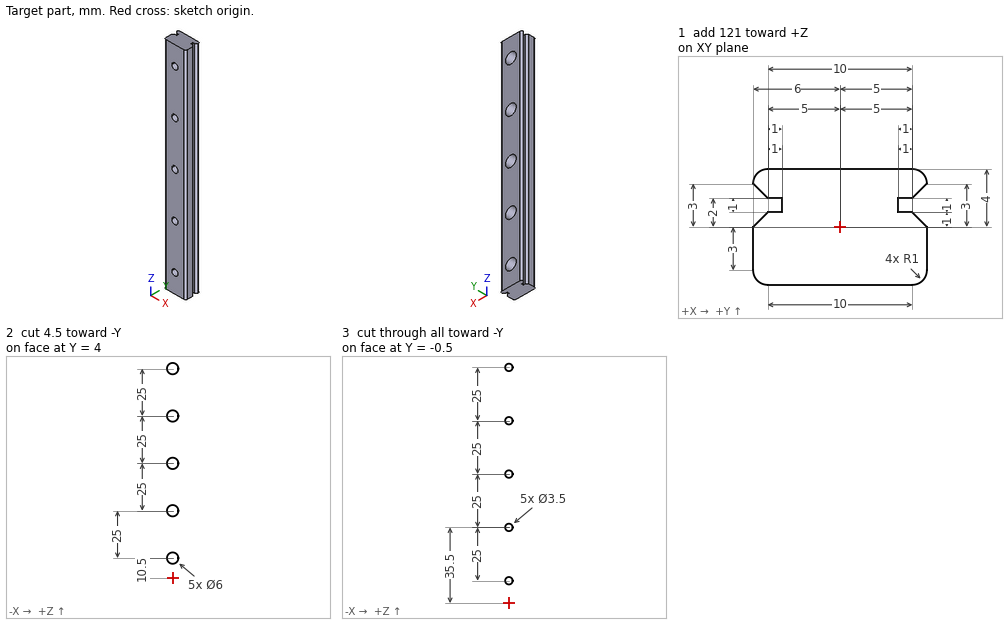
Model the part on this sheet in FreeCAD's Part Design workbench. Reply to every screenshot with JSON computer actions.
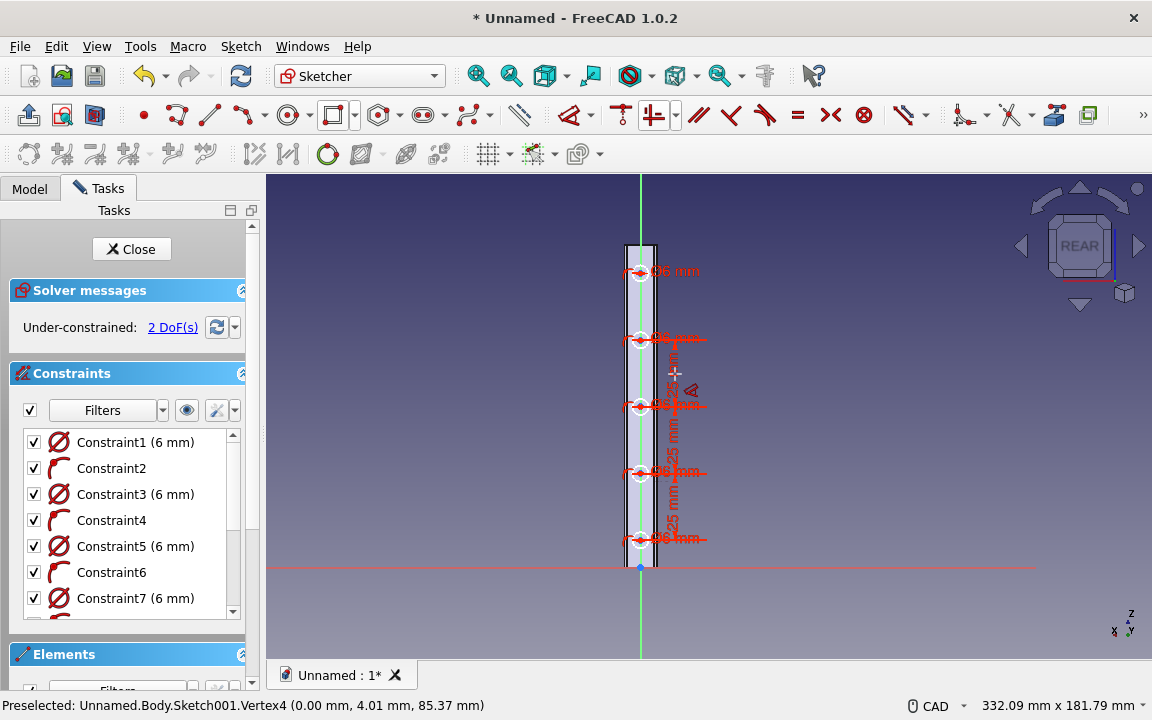
{"action": "left_click", "coordinate": [641, 340]}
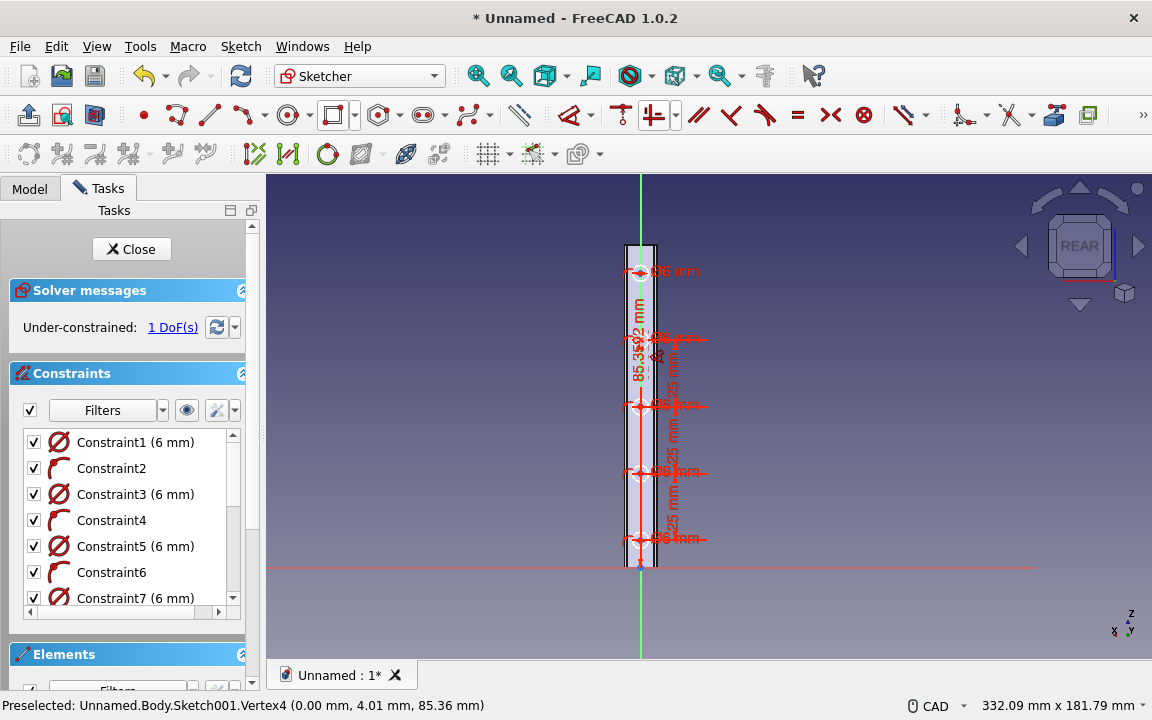
{"action": "left_click", "coordinate": [641, 273]}
{"action": "left_click", "coordinate": [675, 307]}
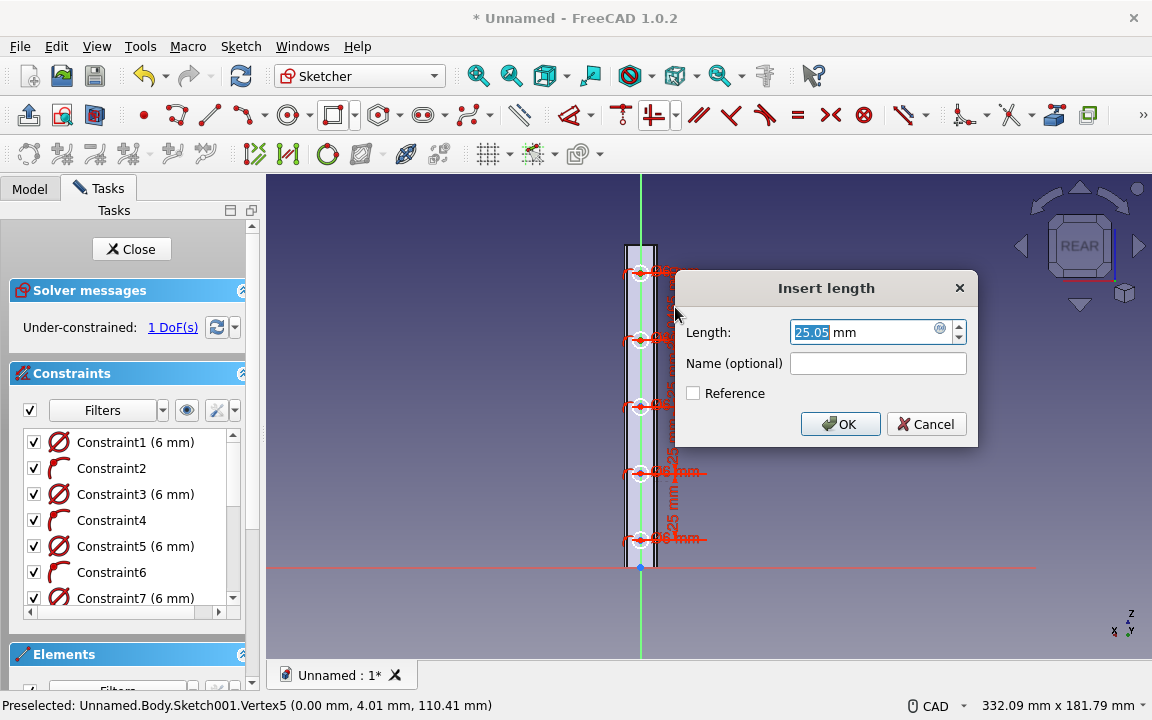
{"action": "type", "text": "25"}
{"action": "key", "text": "Return"}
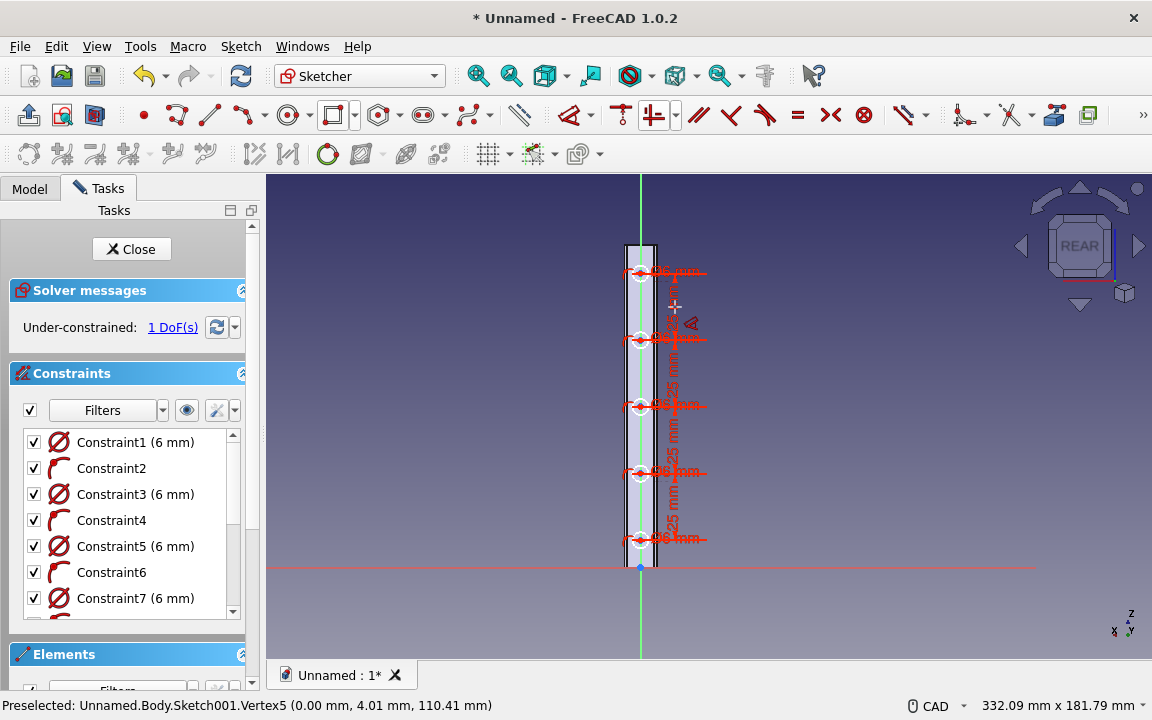
{"action": "scroll", "coordinate": [641, 540], "scroll_direction": "up", "scroll_amount": 2}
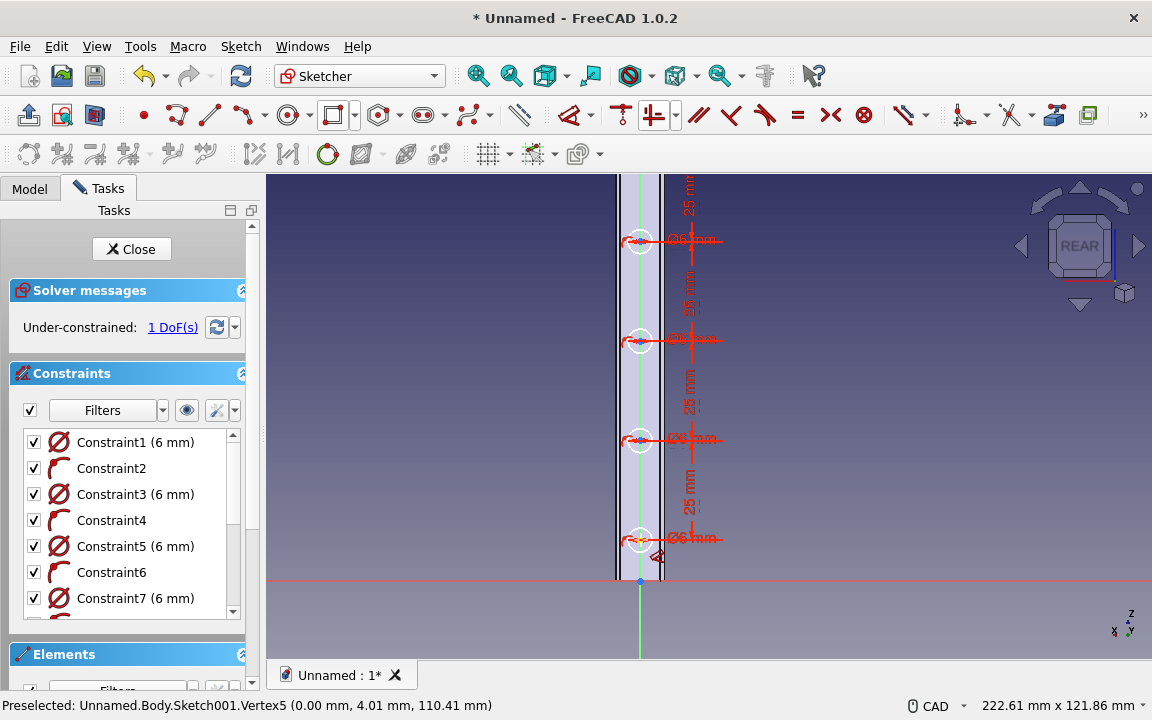
{"action": "left_click", "coordinate": [640, 540]}
{"action": "left_click", "coordinate": [674, 561]}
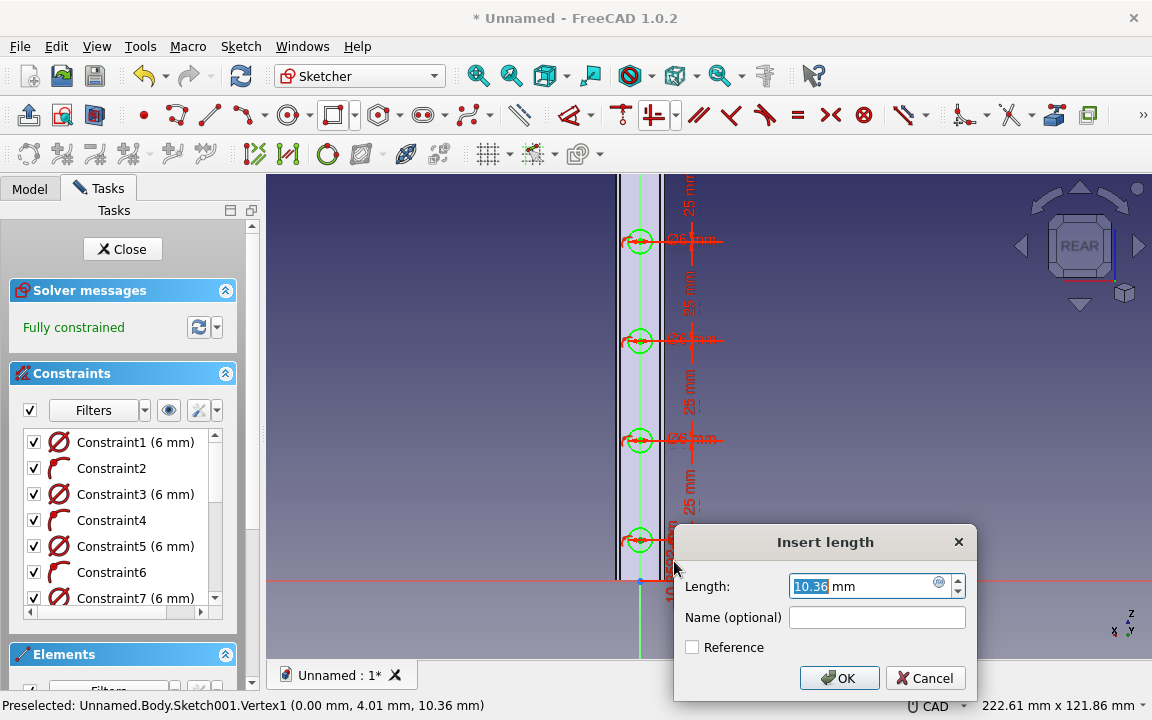
{"action": "type", "text": "10.5"}
{"action": "key", "text": "Return"}
{"action": "key", "text": "Escape"}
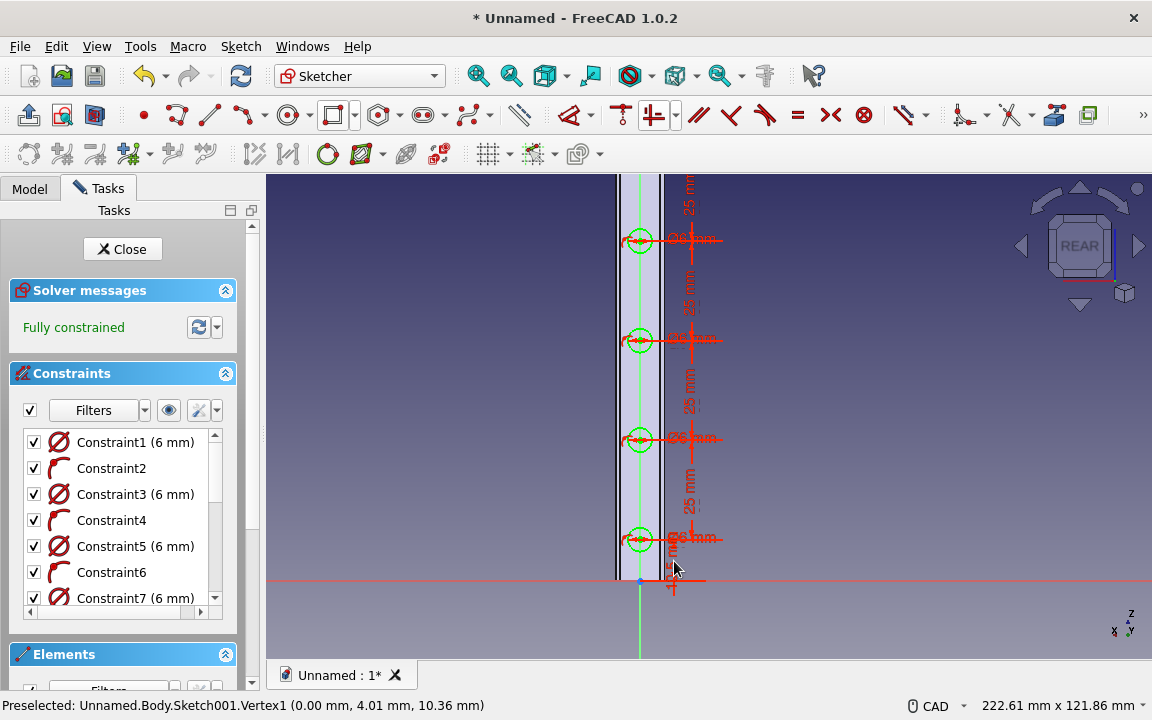
{"action": "left_click", "coordinate": [123, 249]}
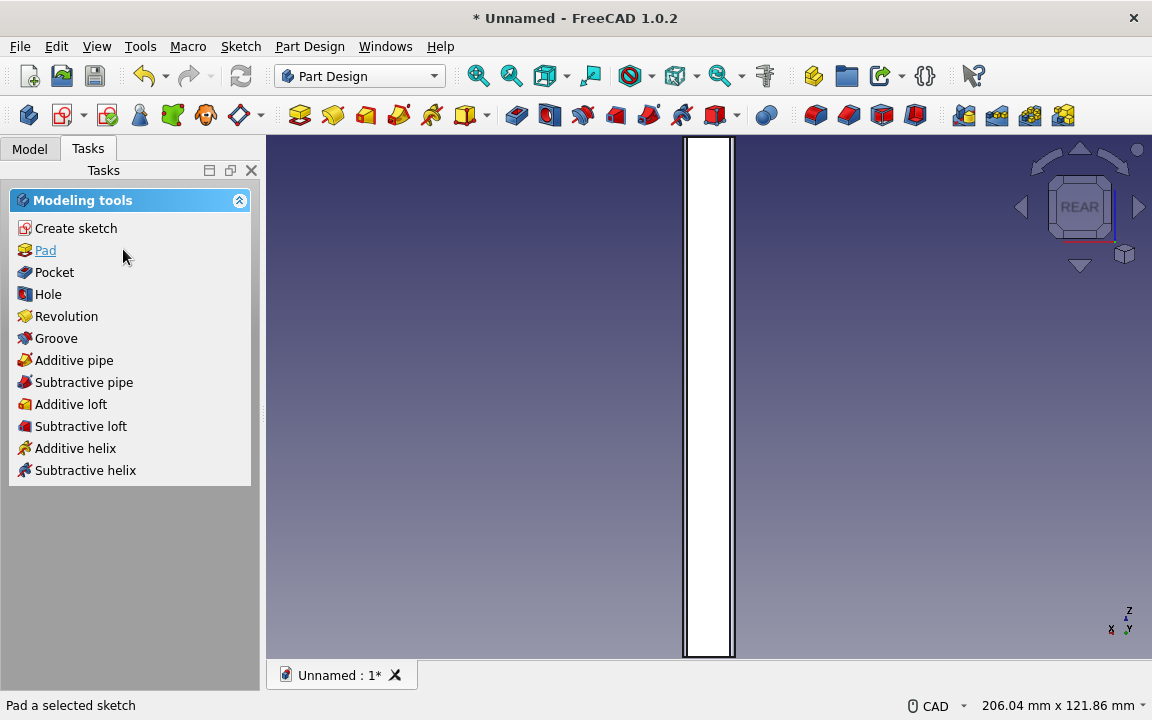
{"action": "left_click", "coordinate": [517, 116]}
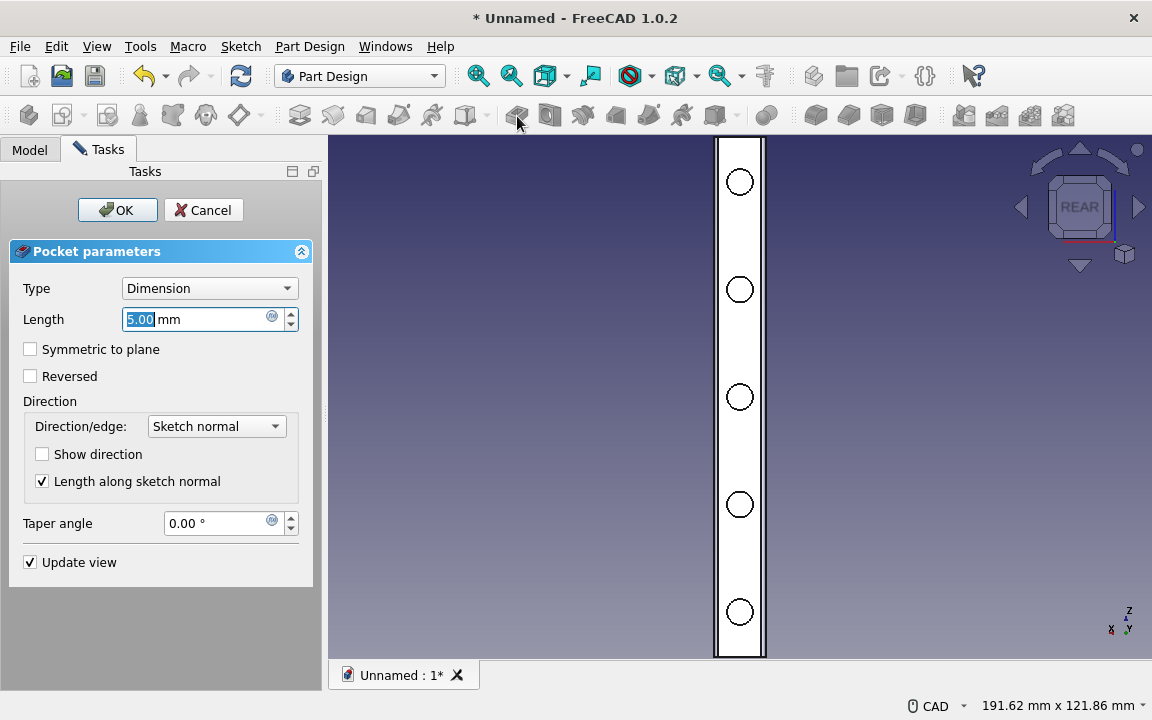
{"action": "type", "text": "4.5"}
{"action": "key", "text": "Tab"}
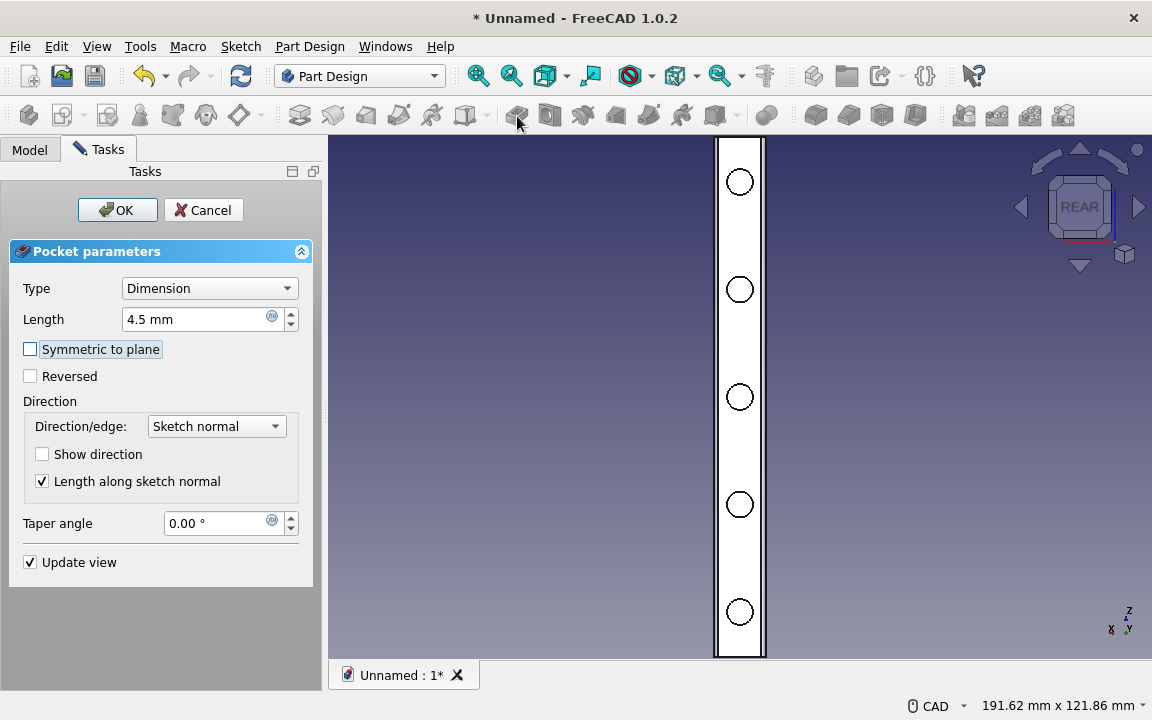
{"action": "left_click", "coordinate": [118, 210]}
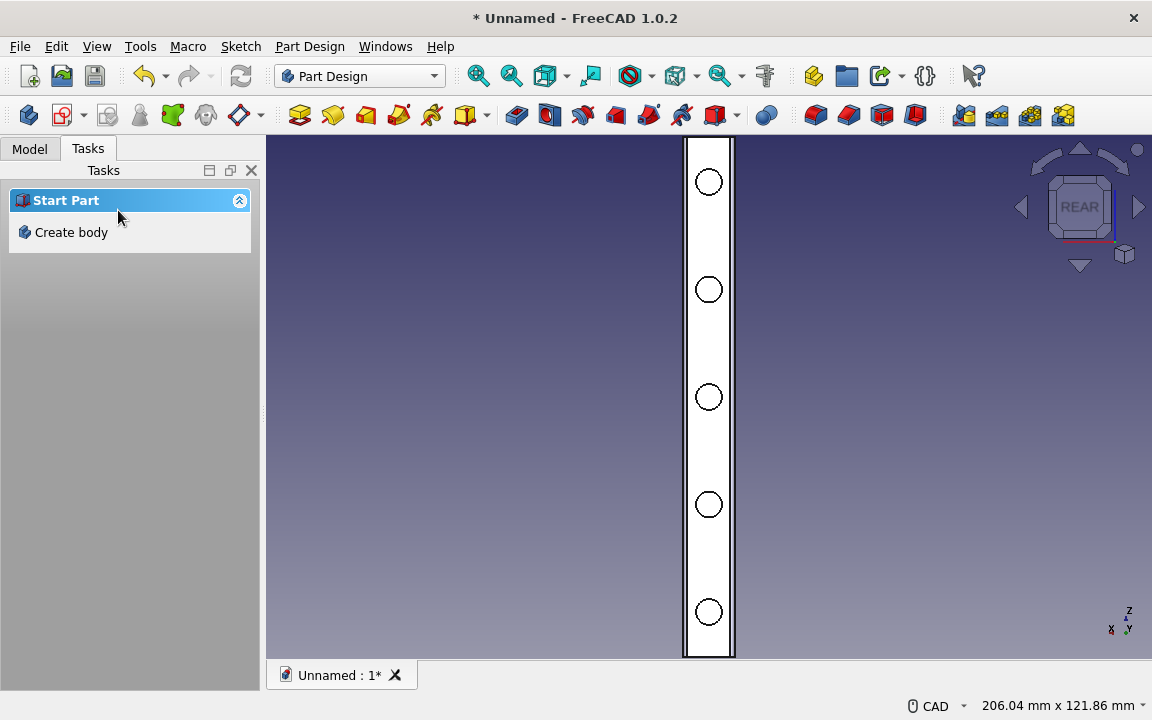
{"action": "left_click", "coordinate": [709, 396]}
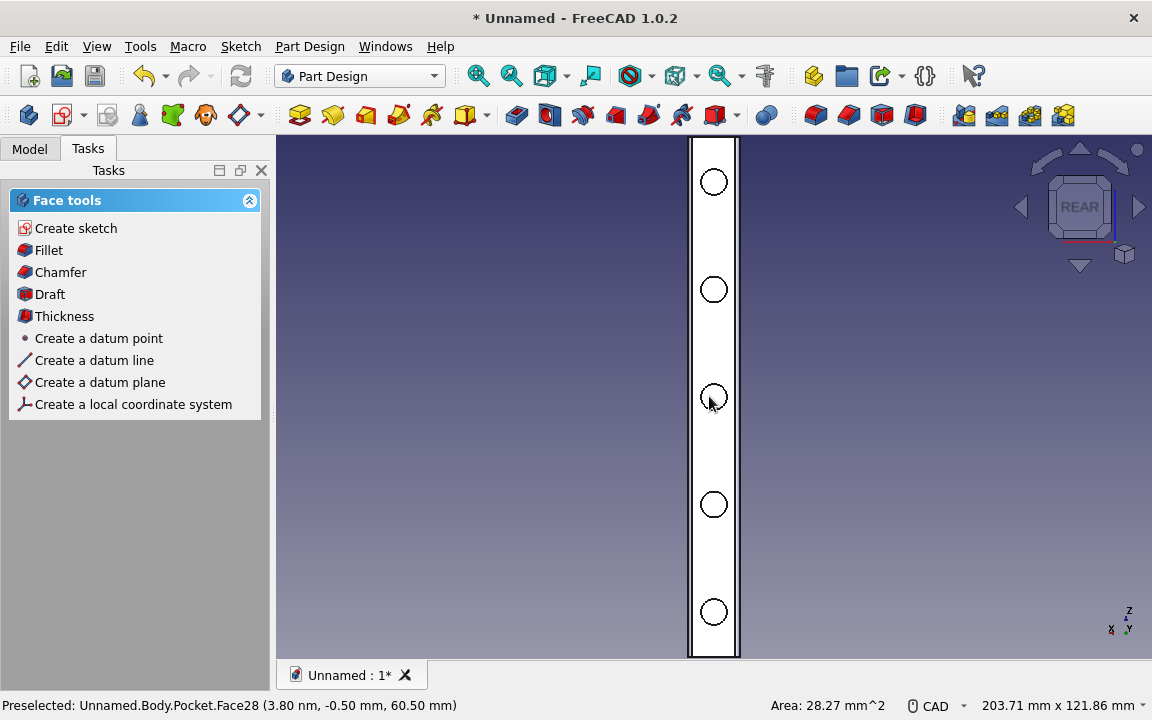
{"action": "left_click", "coordinate": [62, 116]}